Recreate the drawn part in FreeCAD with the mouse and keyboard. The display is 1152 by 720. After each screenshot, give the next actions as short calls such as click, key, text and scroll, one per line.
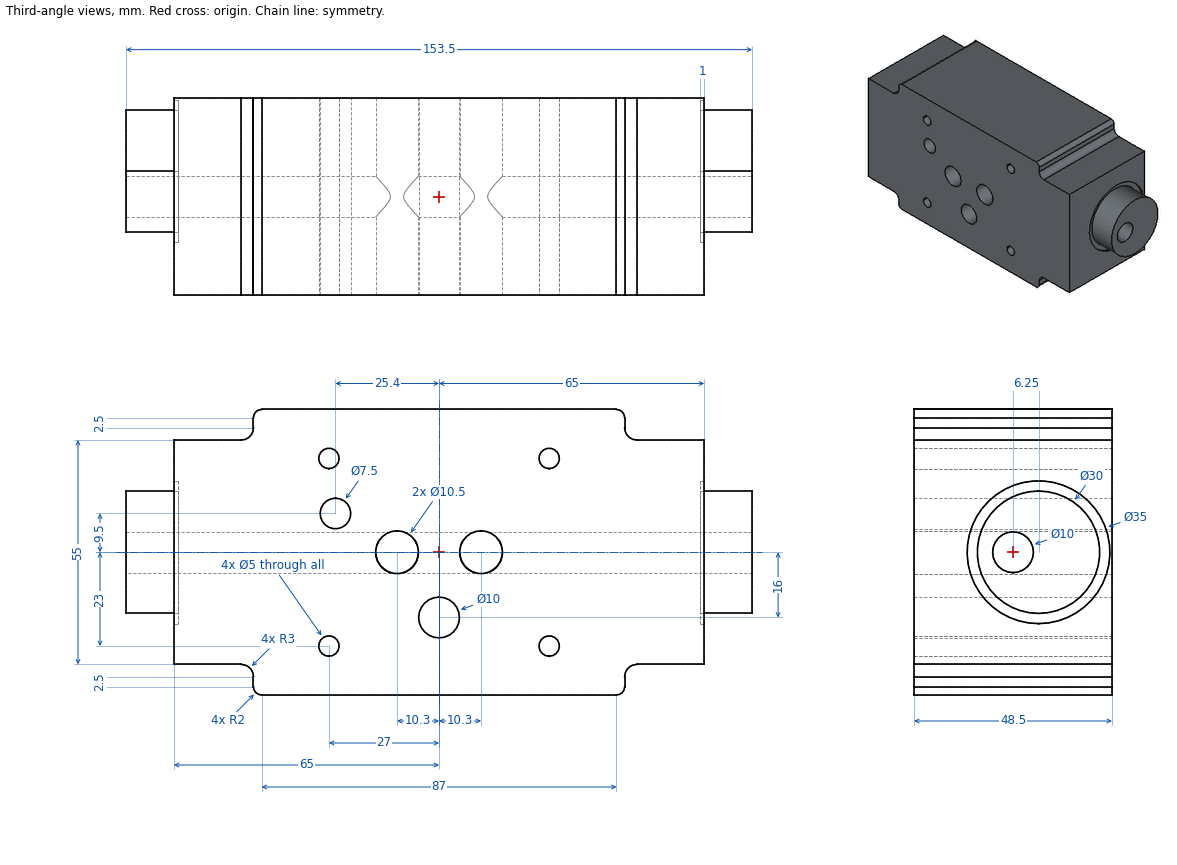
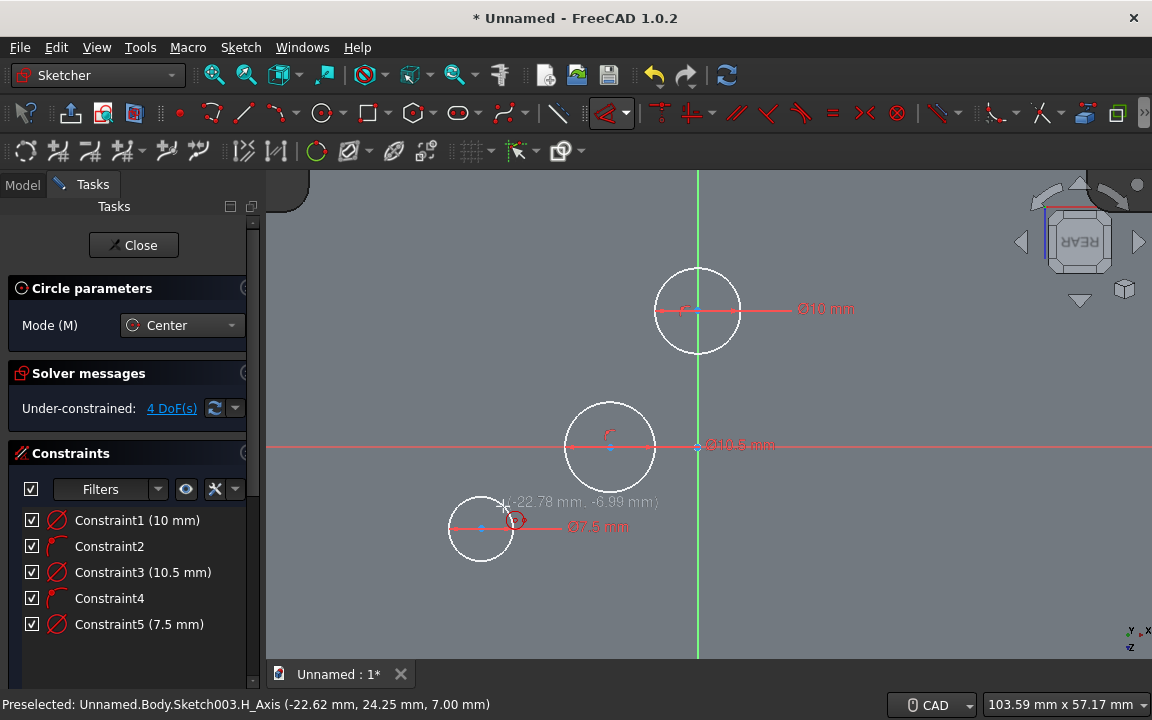
click(786, 447)
move(818, 415)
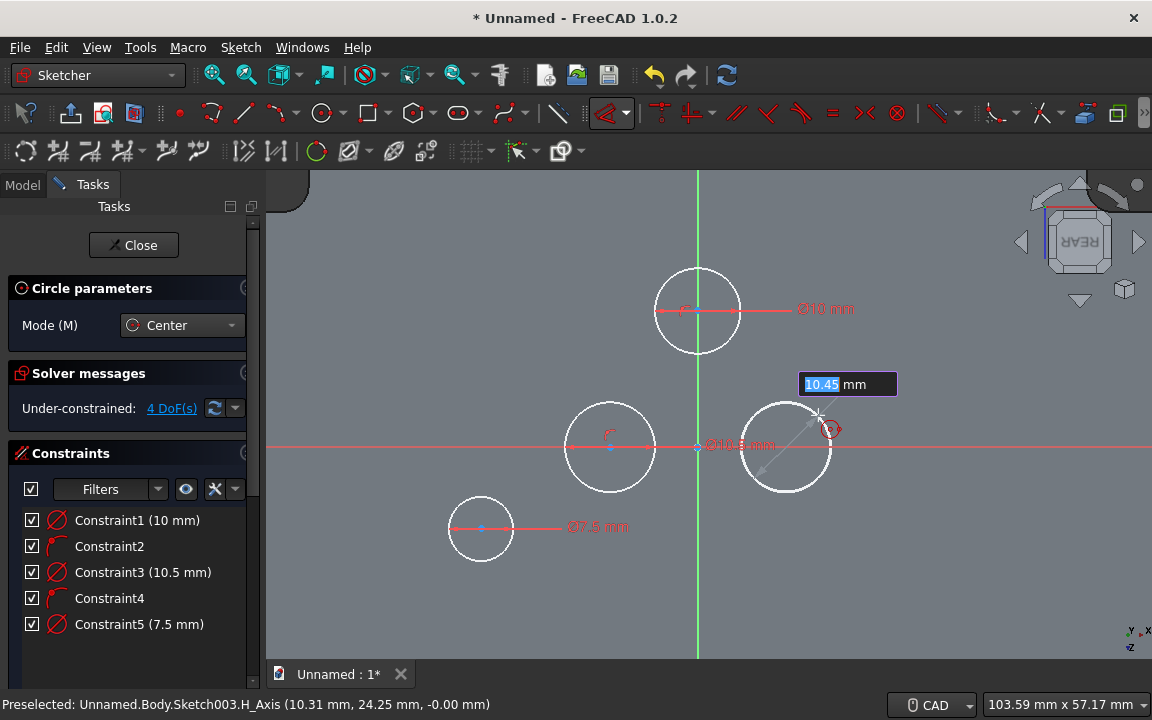
text(10.5)
key(Return)
key(Escape)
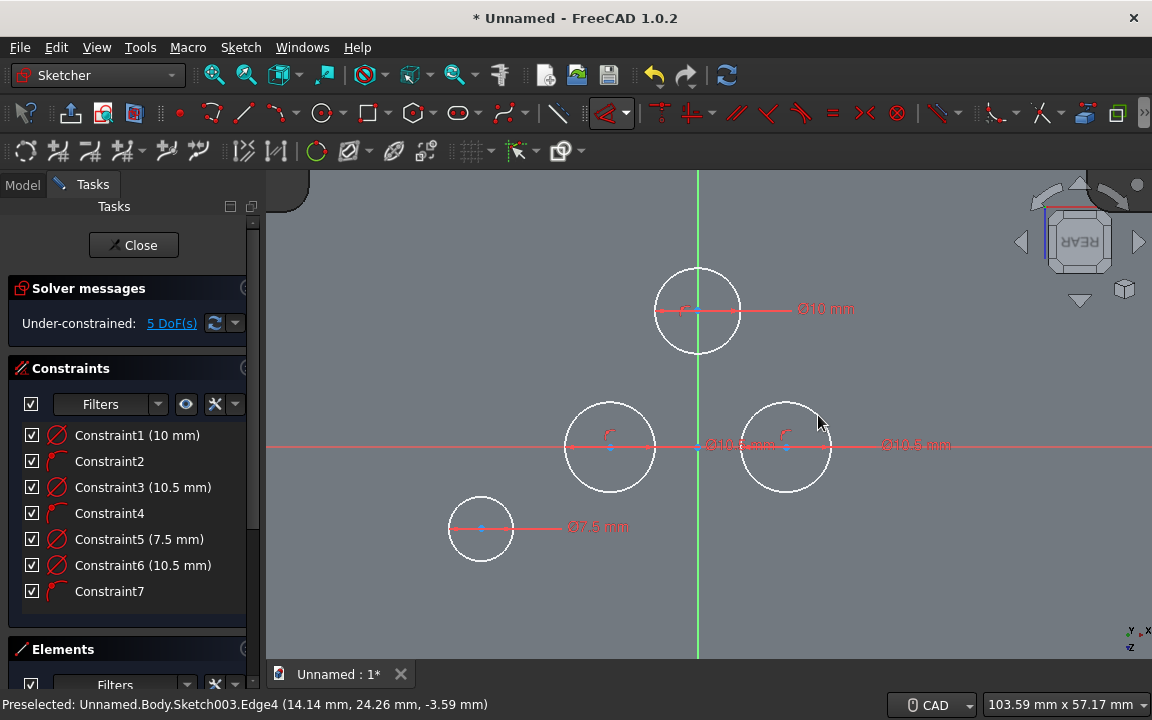
click(698, 311)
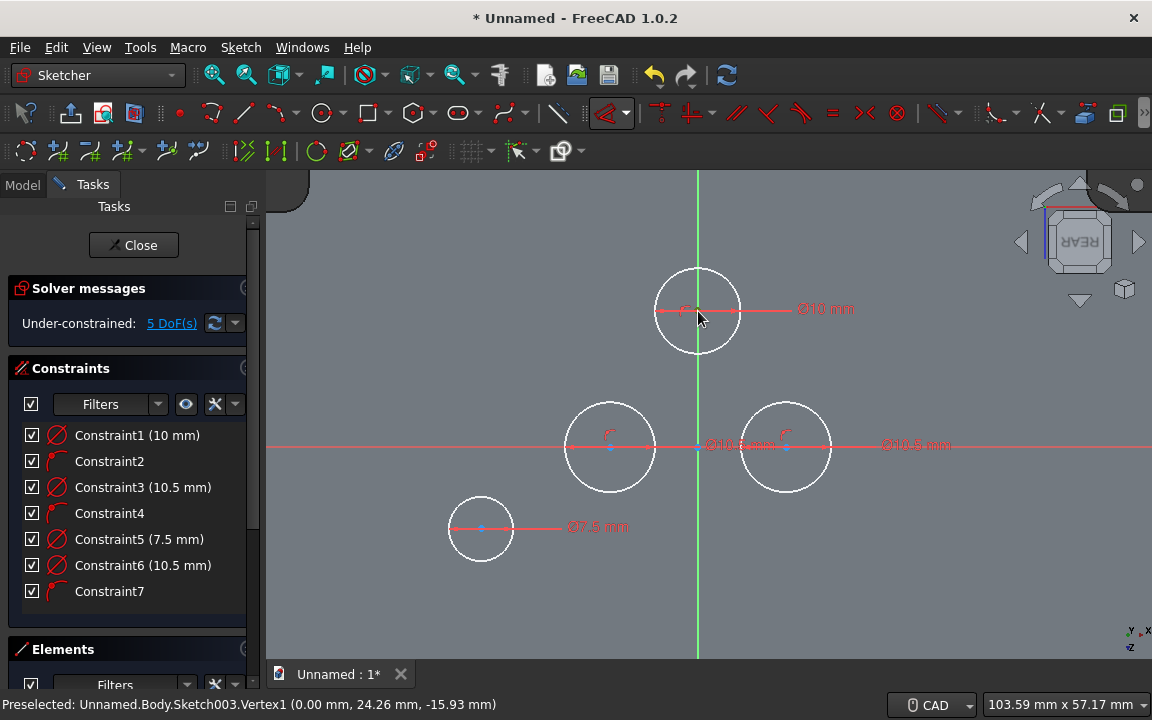
click(628, 114)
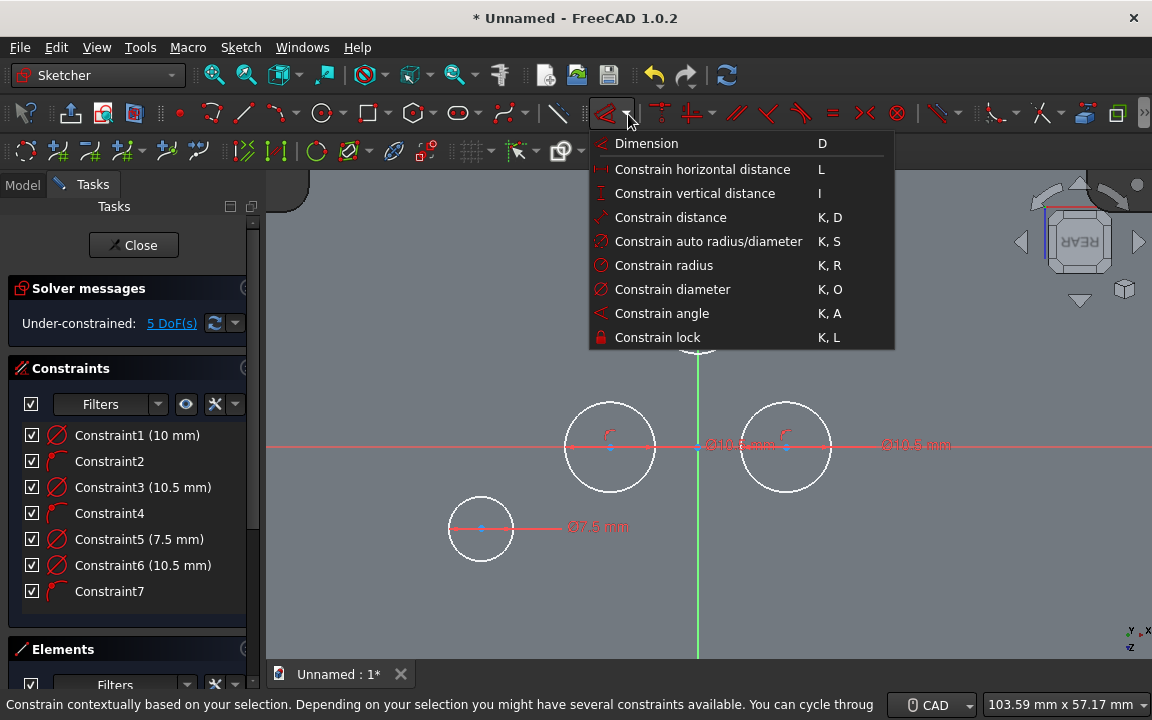
click(742, 193)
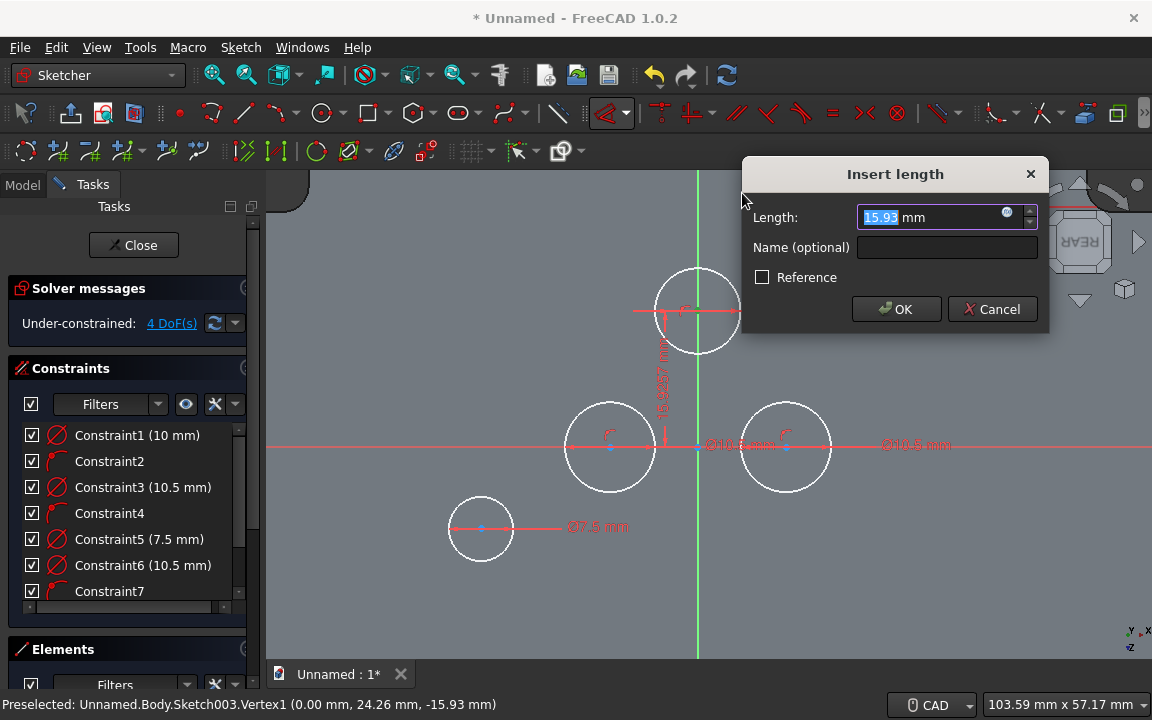
text(16)
key(Return)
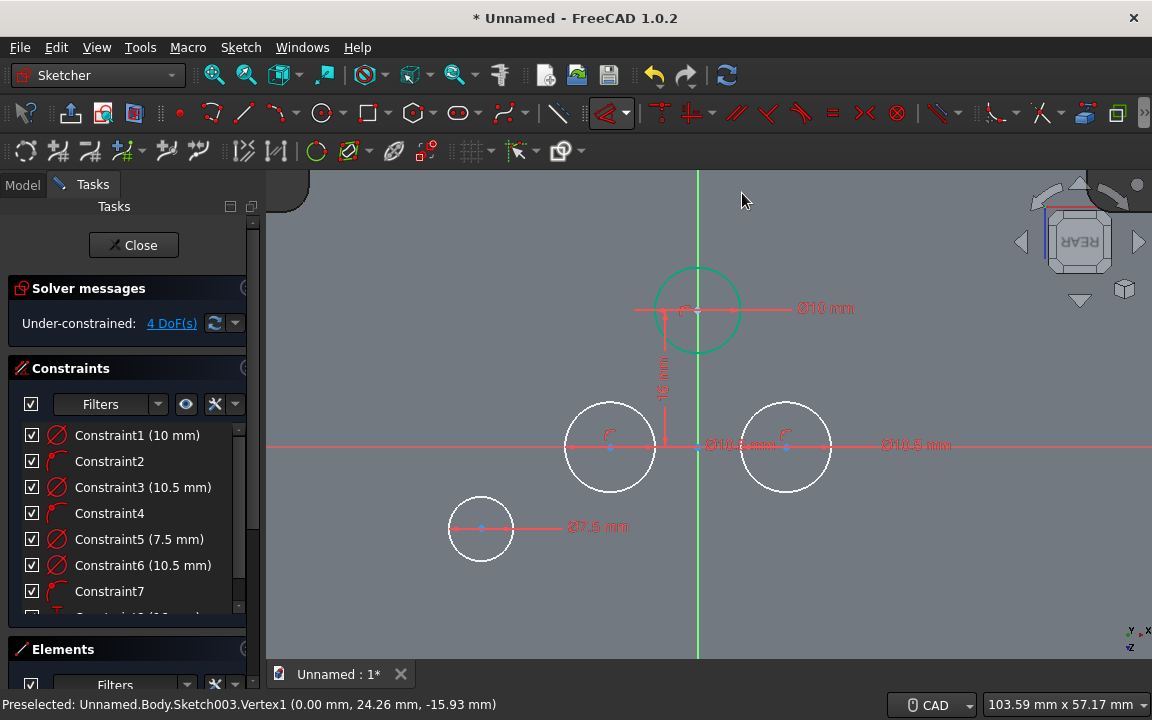
click(481, 529)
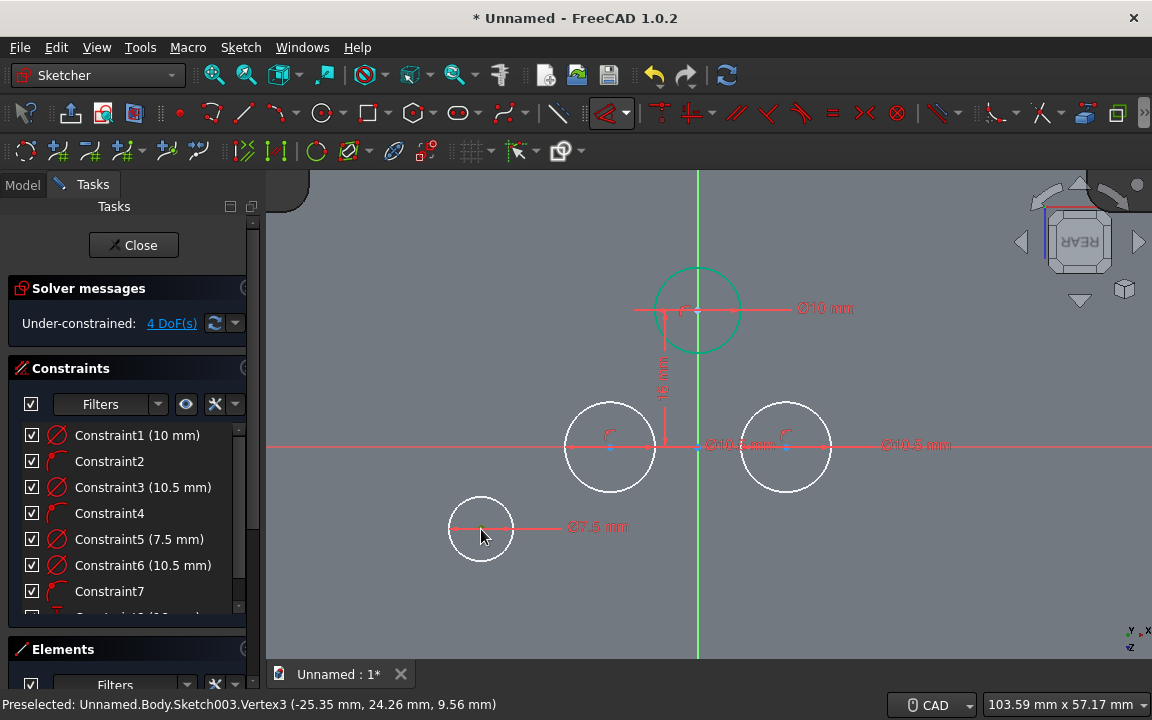
key(i)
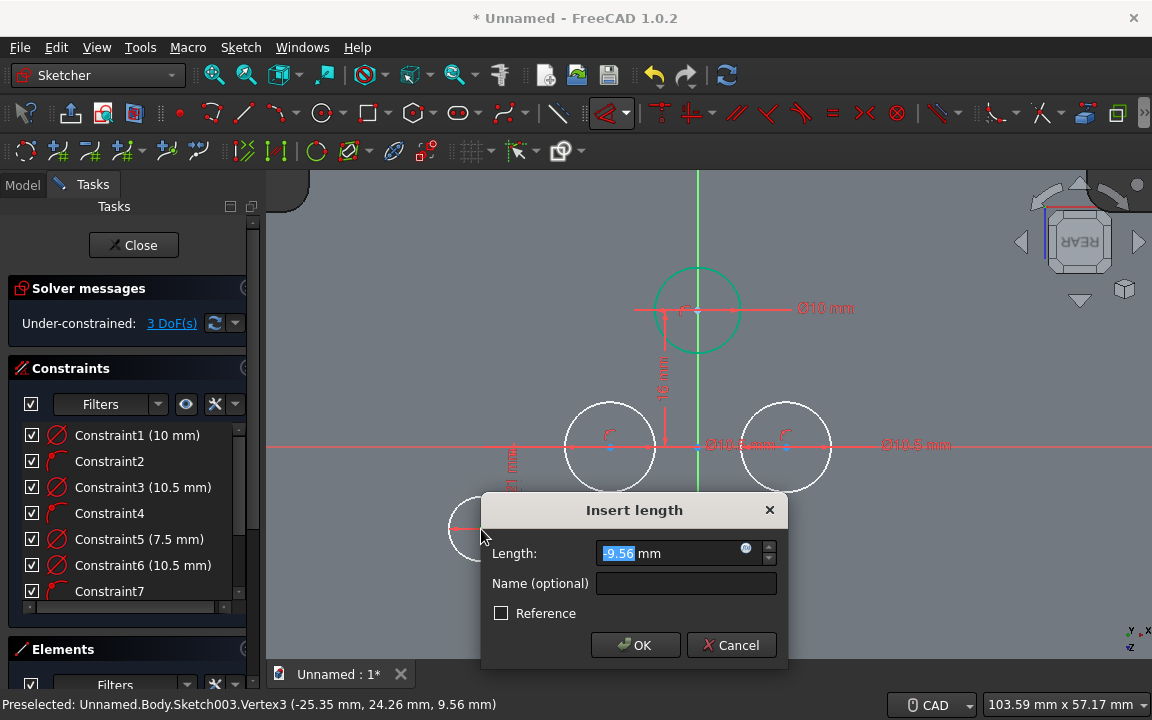
text(-9.5)
key(Return)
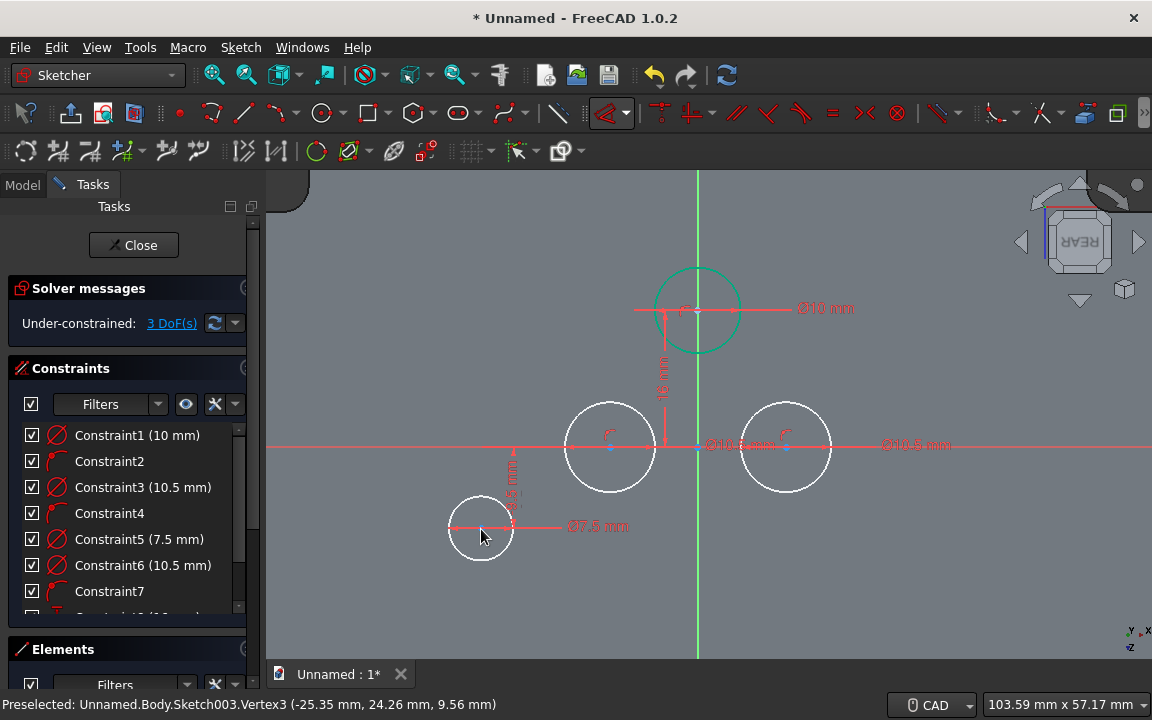
click(610, 447)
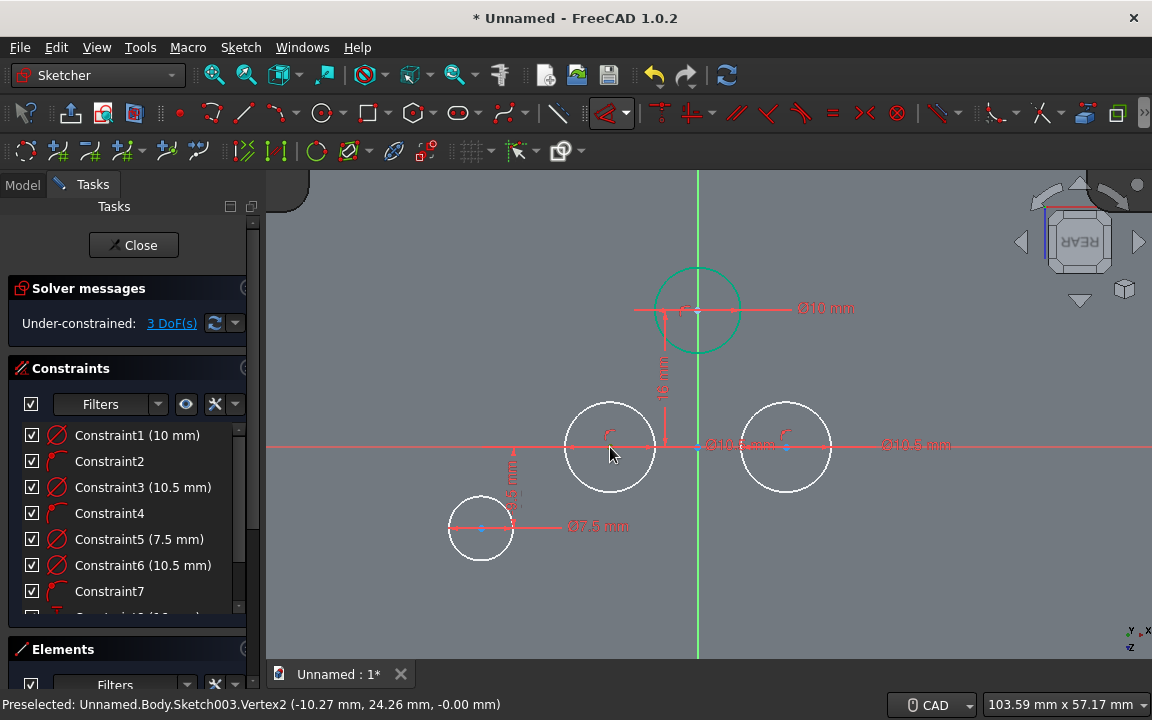
key(l)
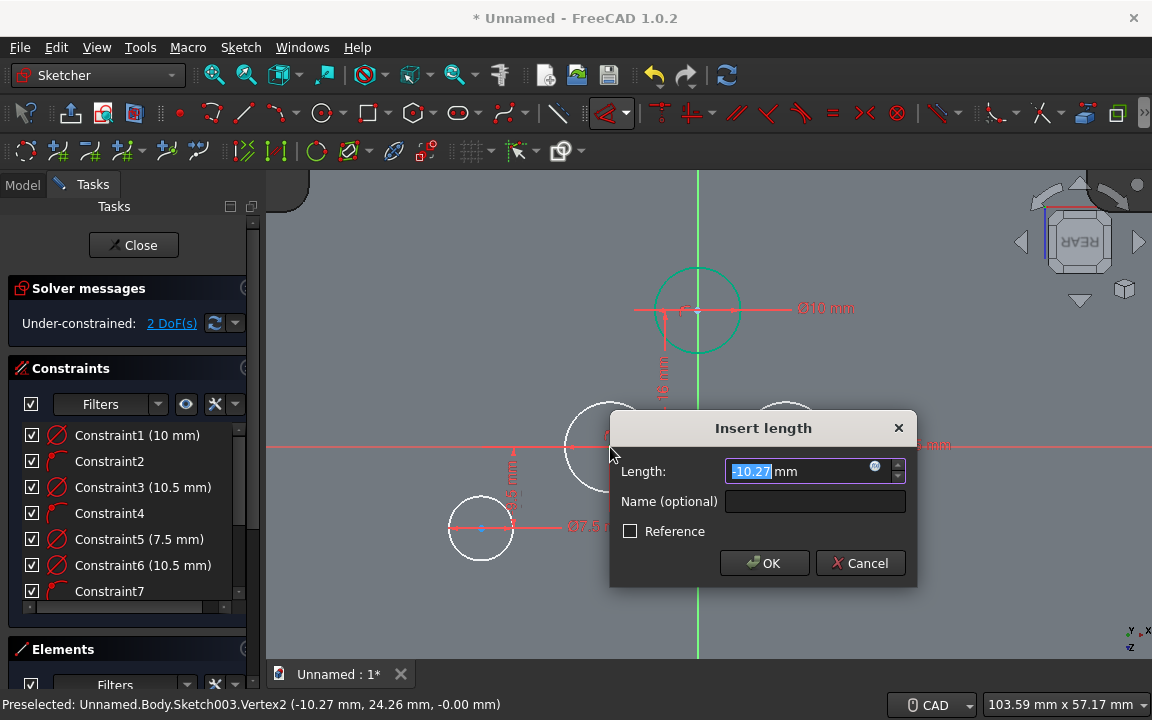
text(-10.3)
key(Return)